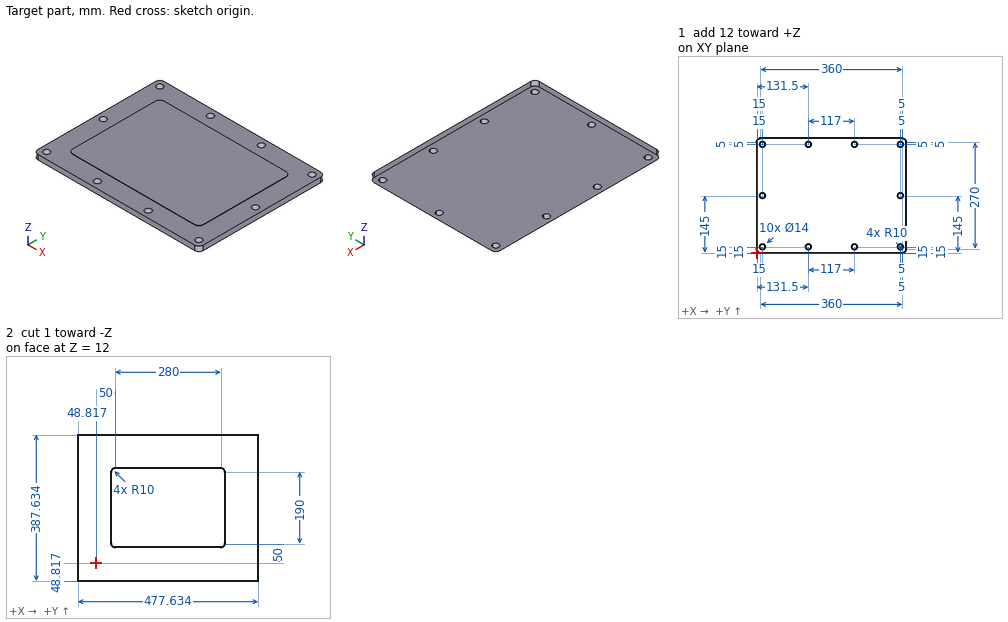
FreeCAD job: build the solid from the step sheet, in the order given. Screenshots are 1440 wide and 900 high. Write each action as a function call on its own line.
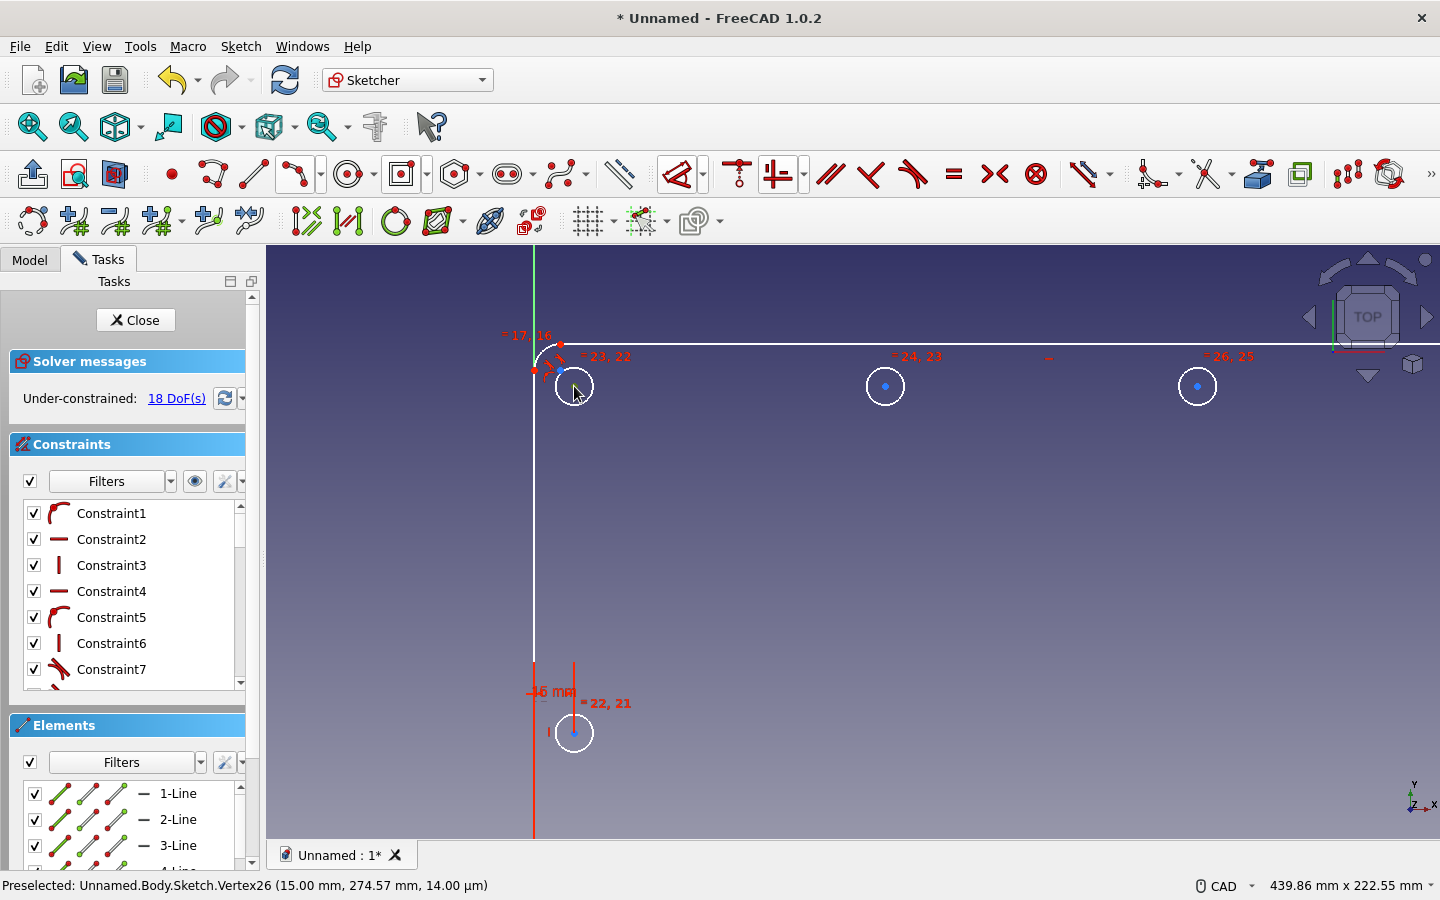
key(l)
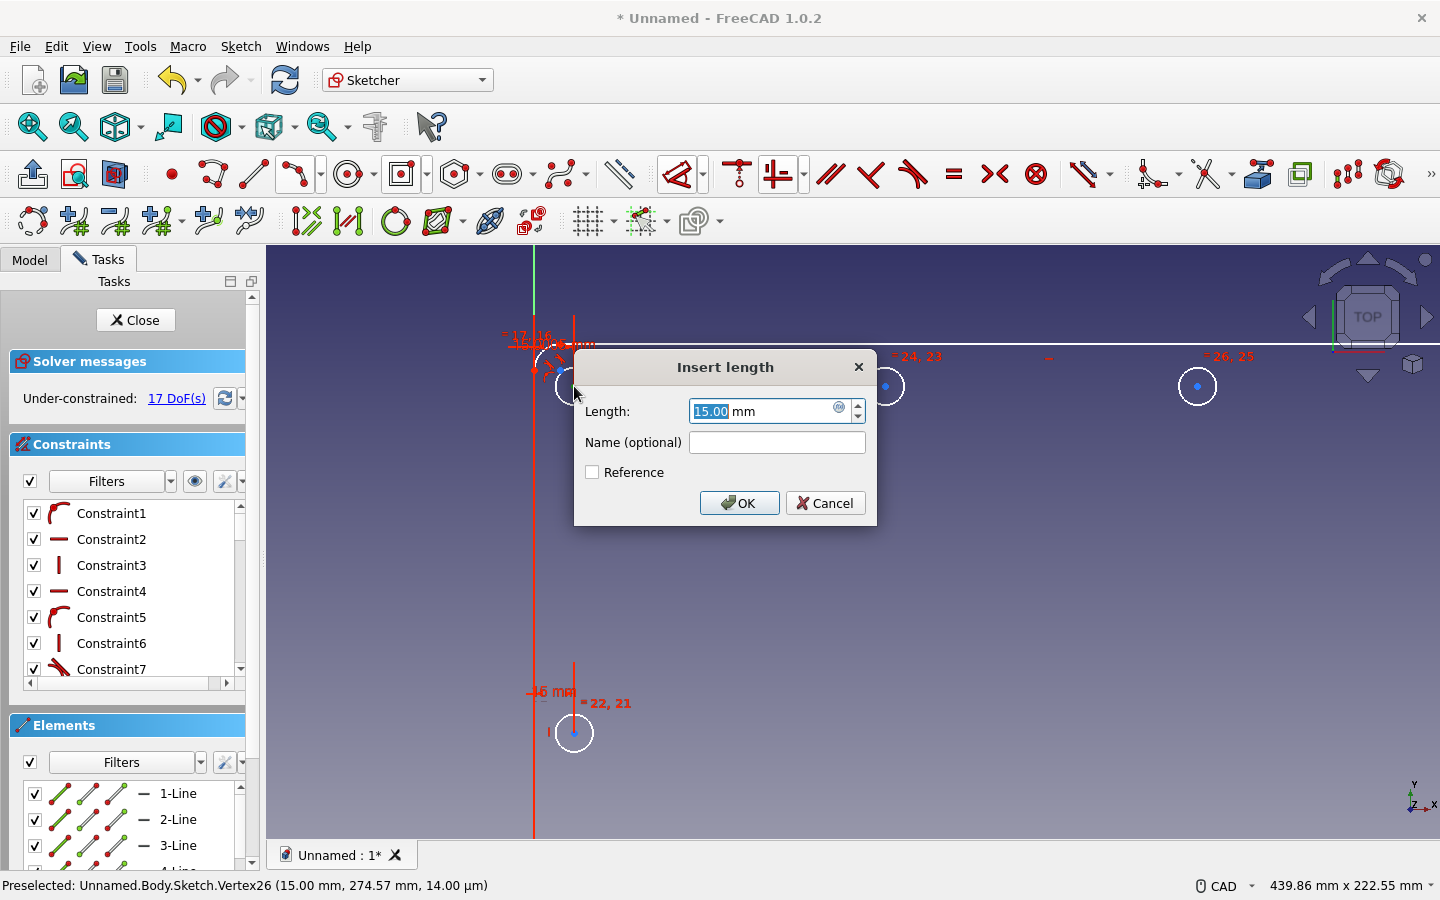
text(15)
key(Return)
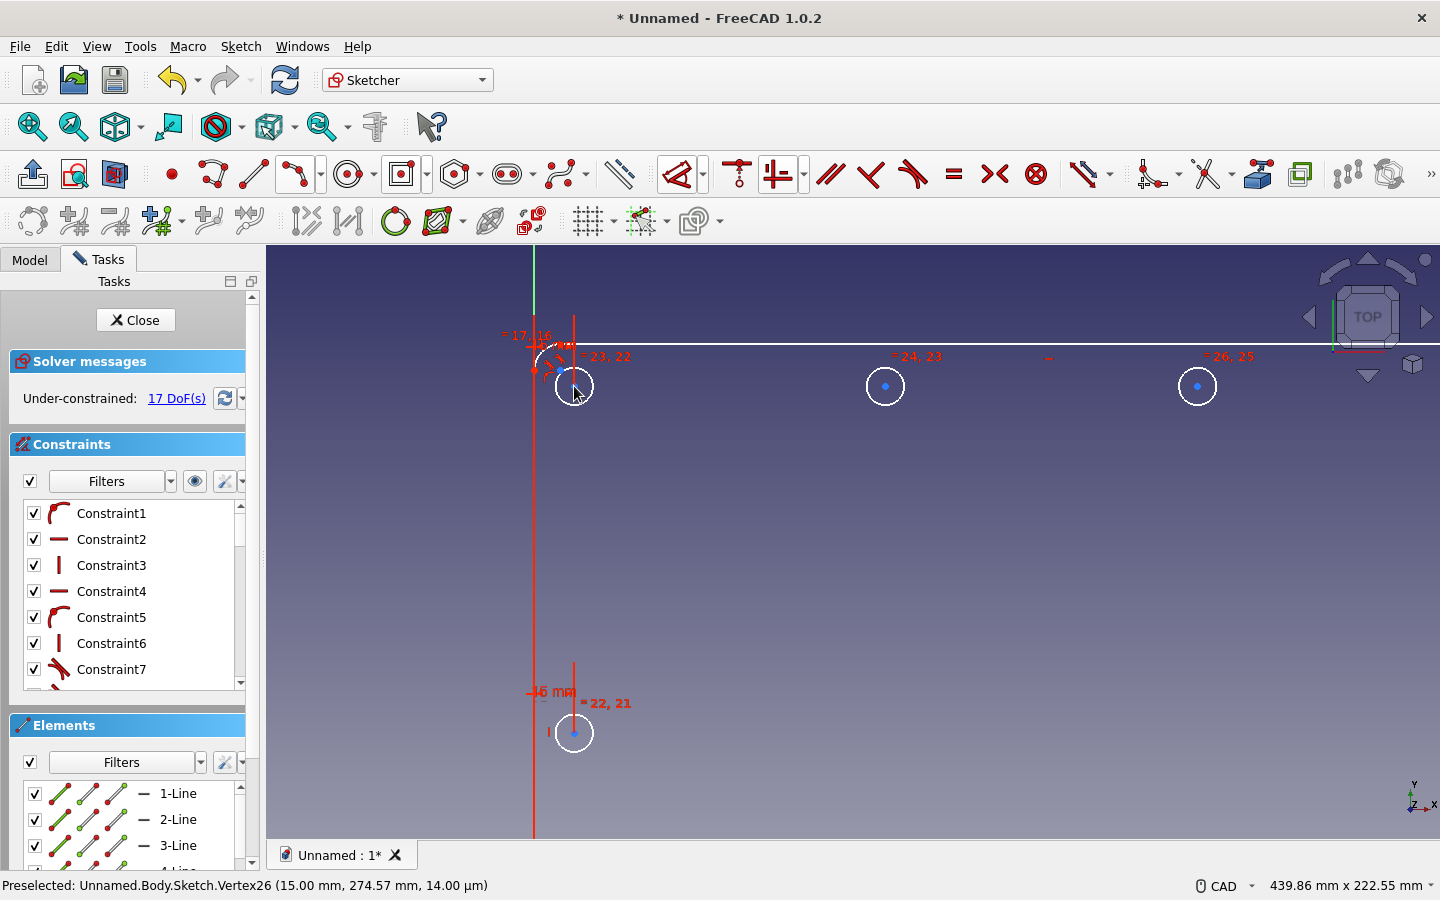
scroll(575, 387, down, 4)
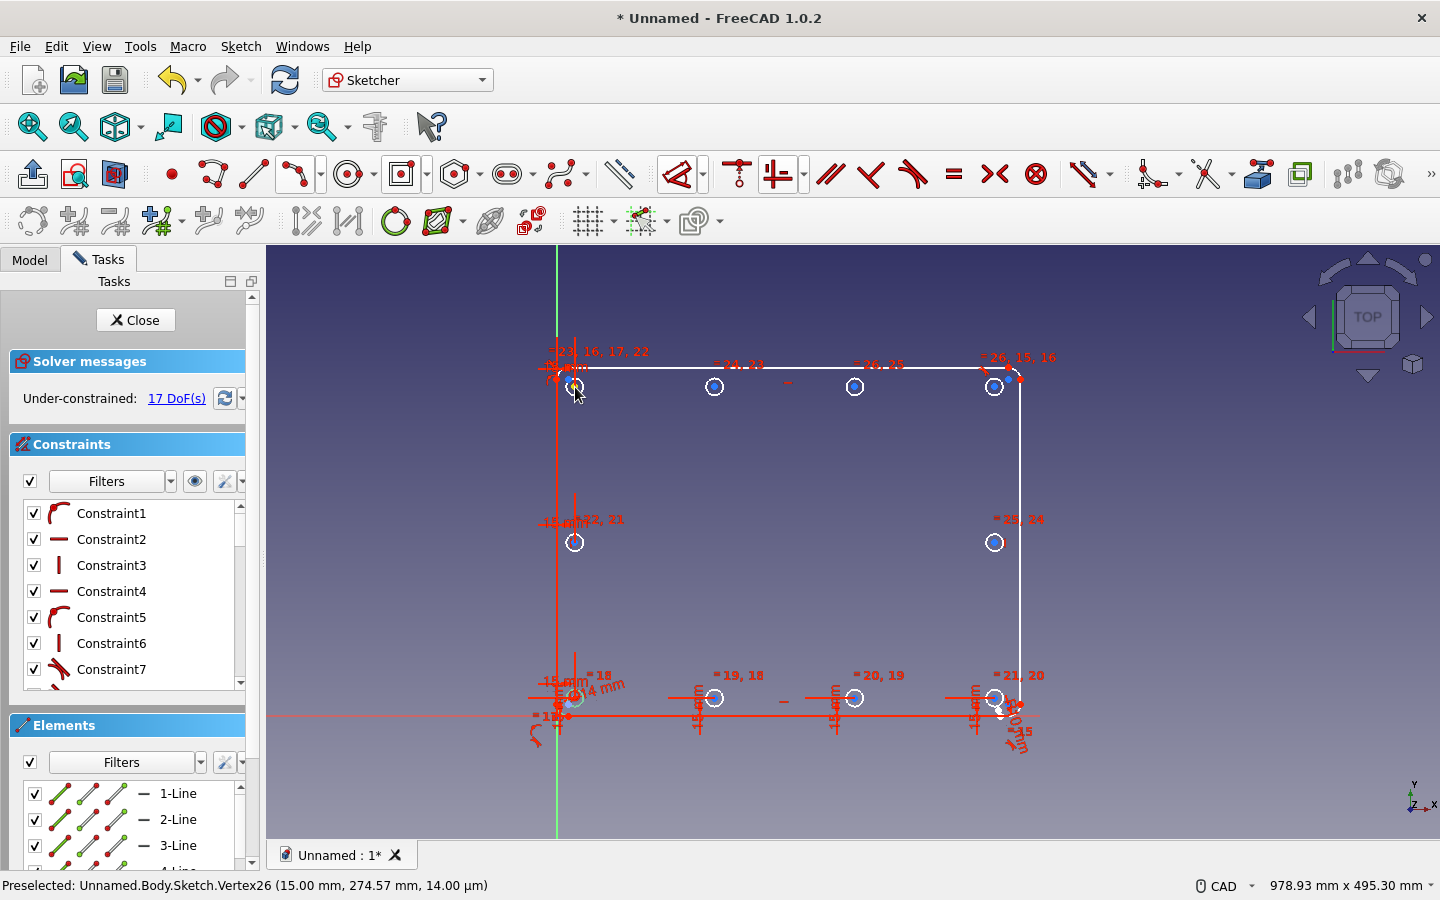
scroll(1001, 716, up, 10)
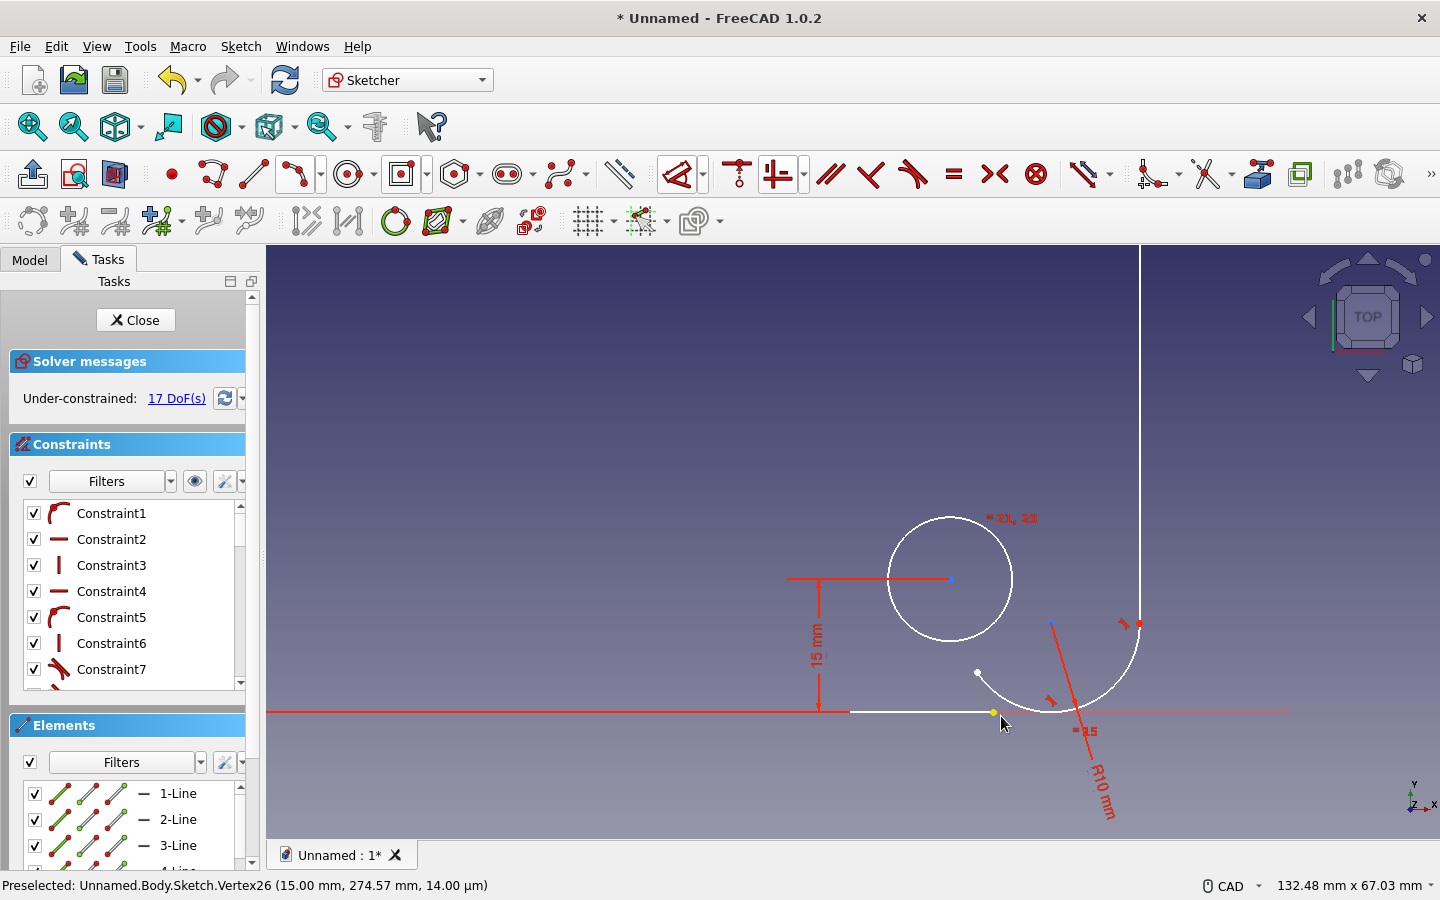
click(994, 712)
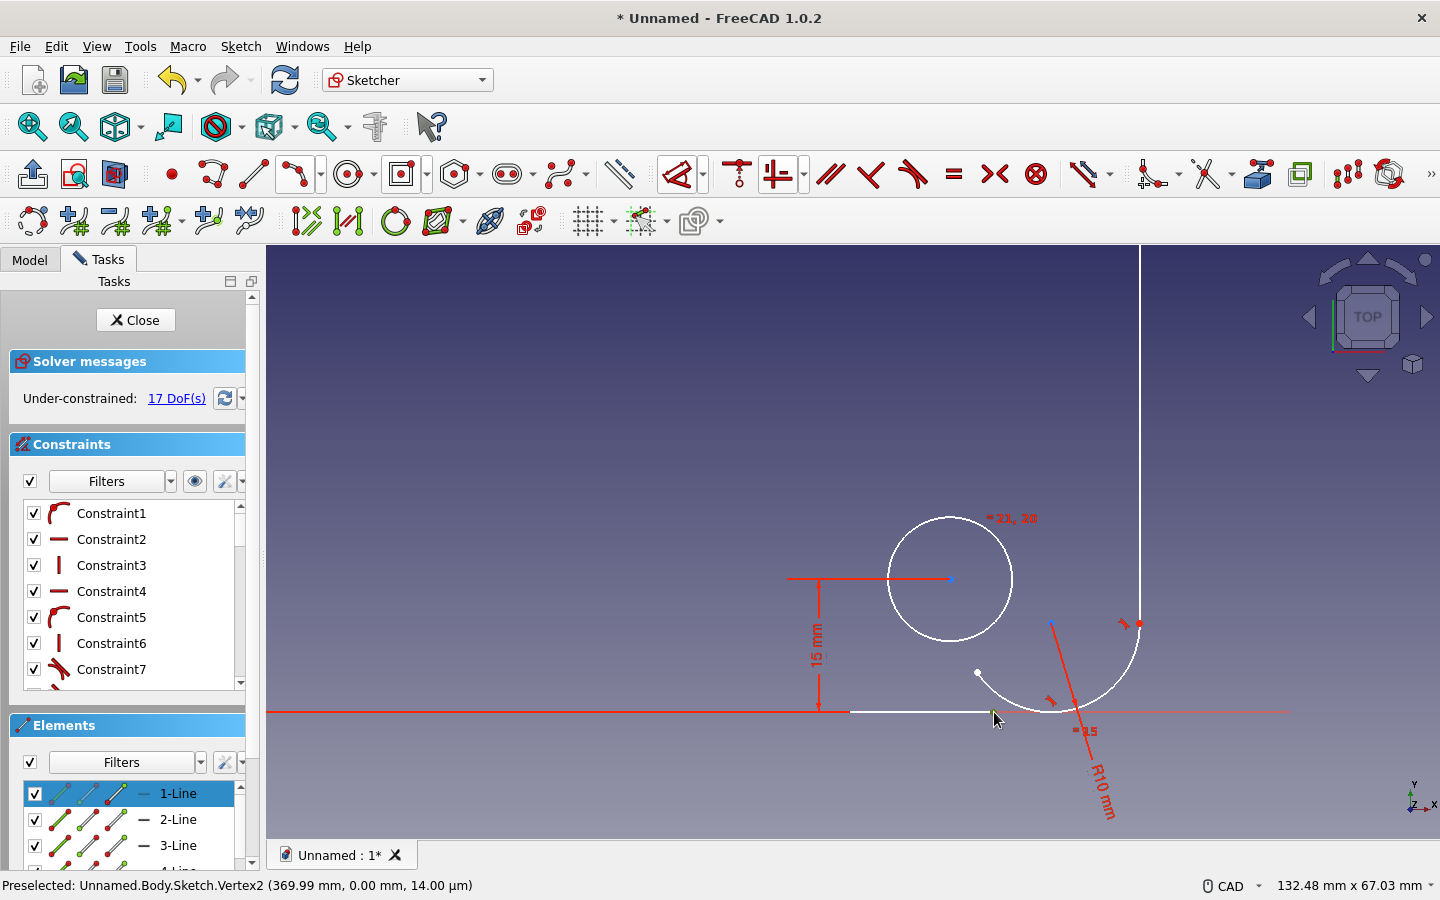
click(950, 579)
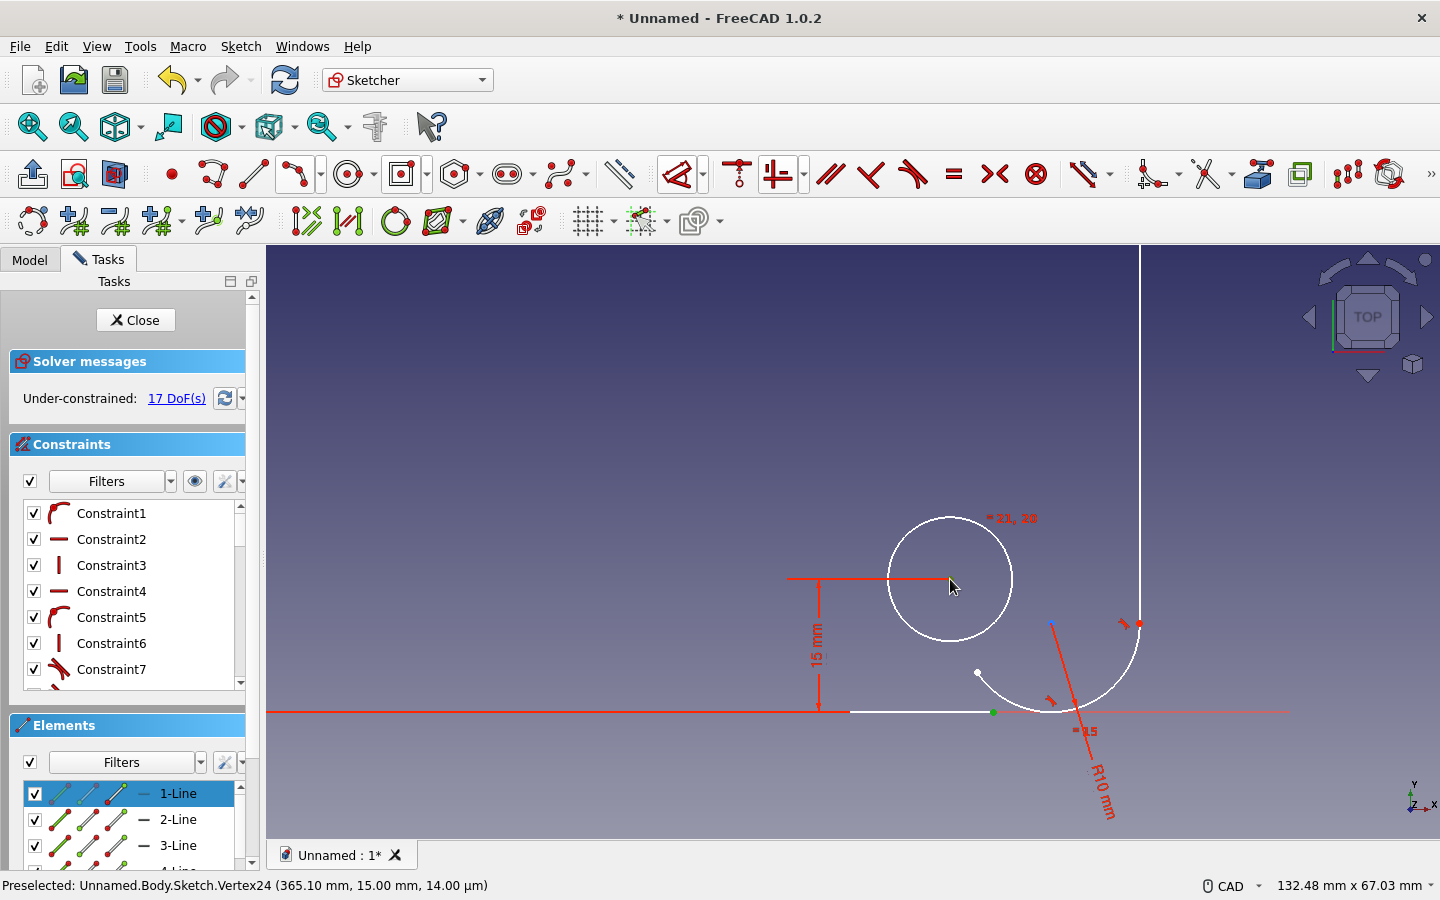
key(l)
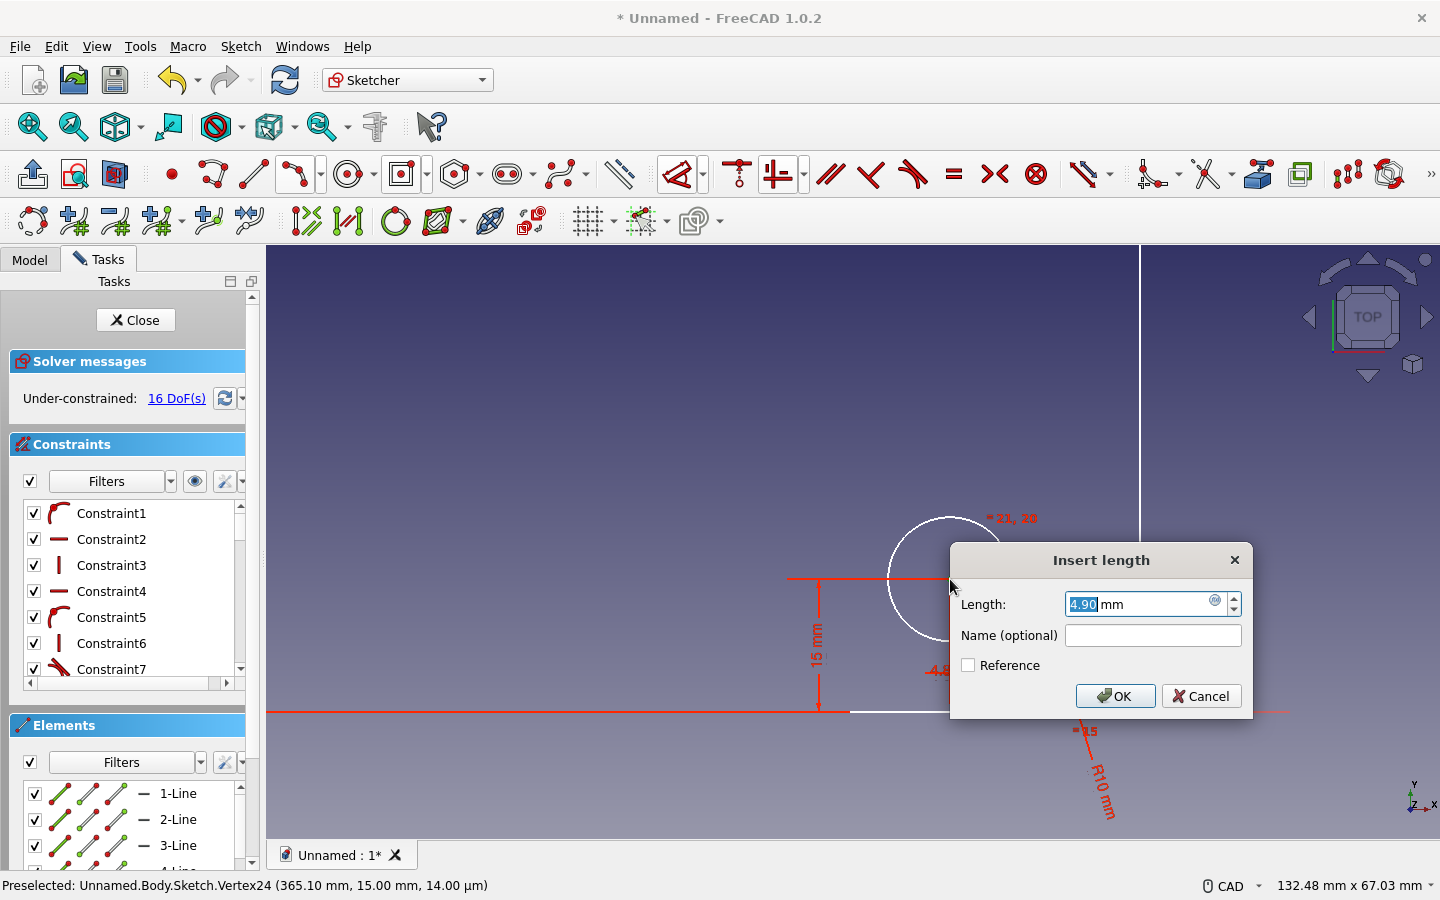
text(5)
key(Return)